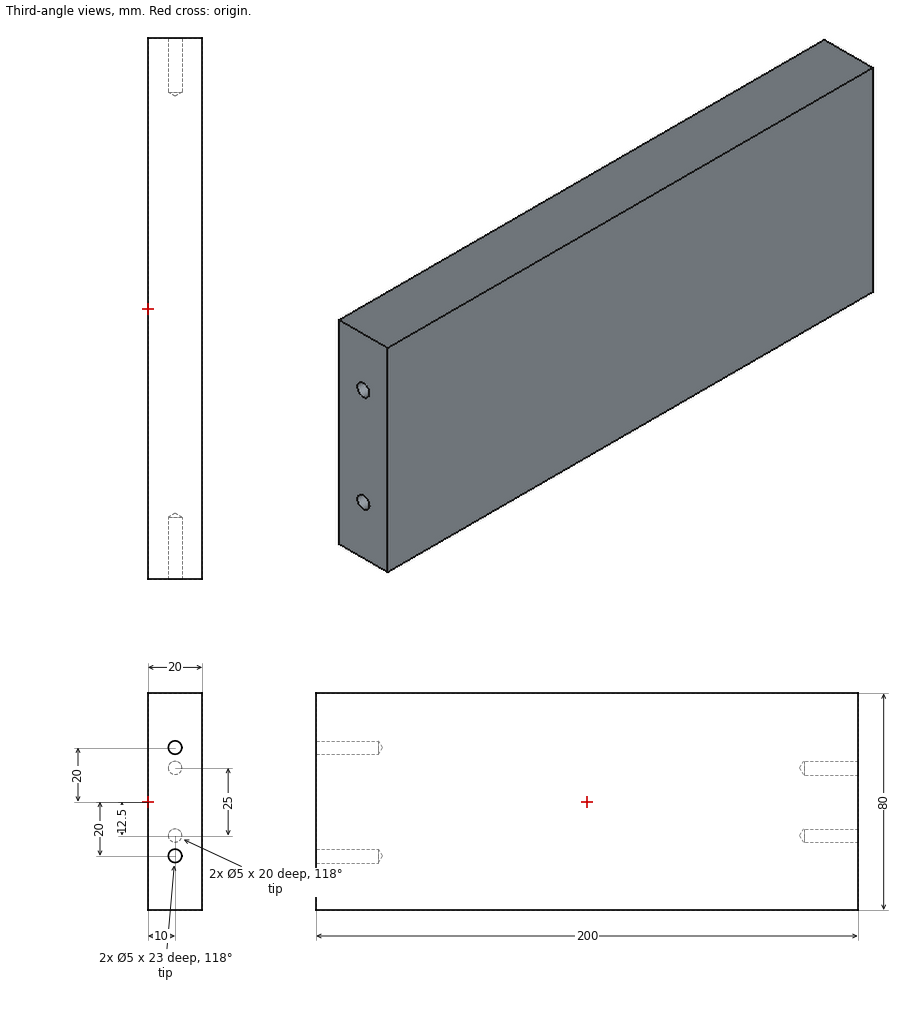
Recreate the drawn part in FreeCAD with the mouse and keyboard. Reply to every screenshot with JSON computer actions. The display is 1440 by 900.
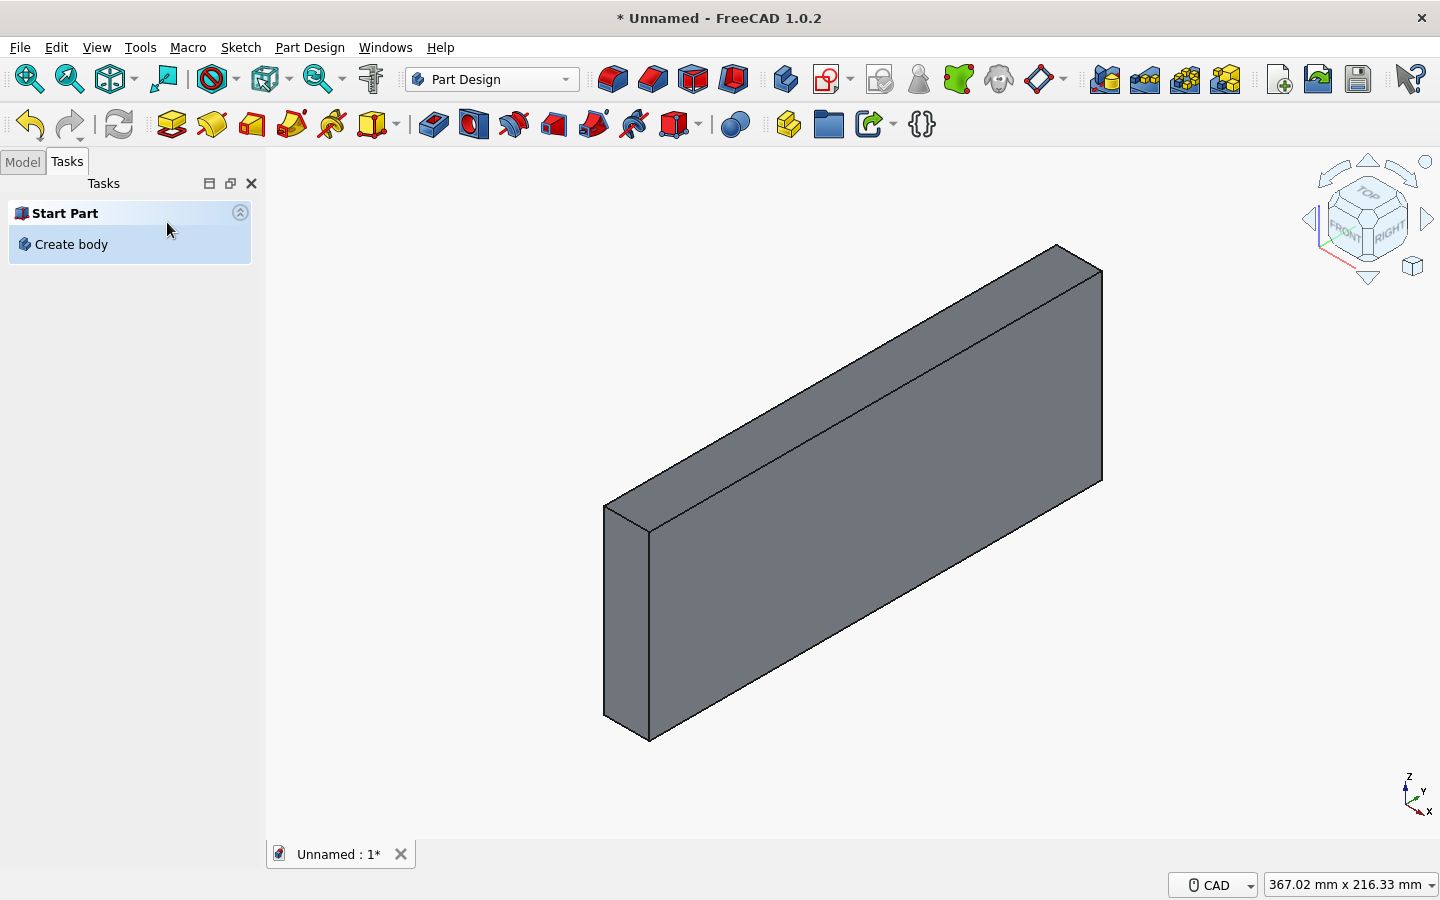
{"action": "left_click", "coordinate": [627, 652]}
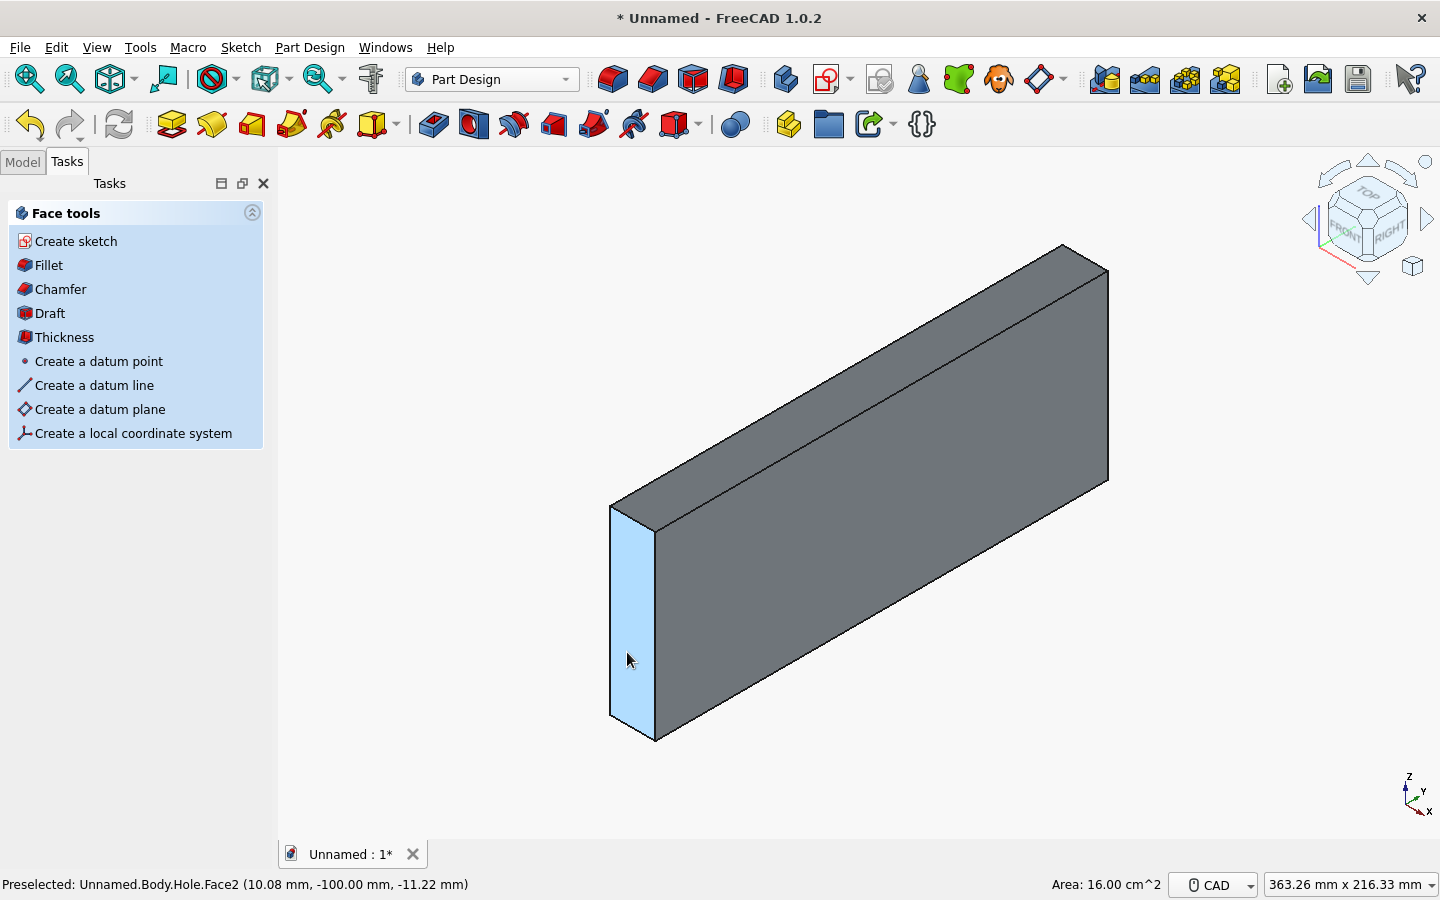
{"action": "left_click", "coordinate": [826, 80]}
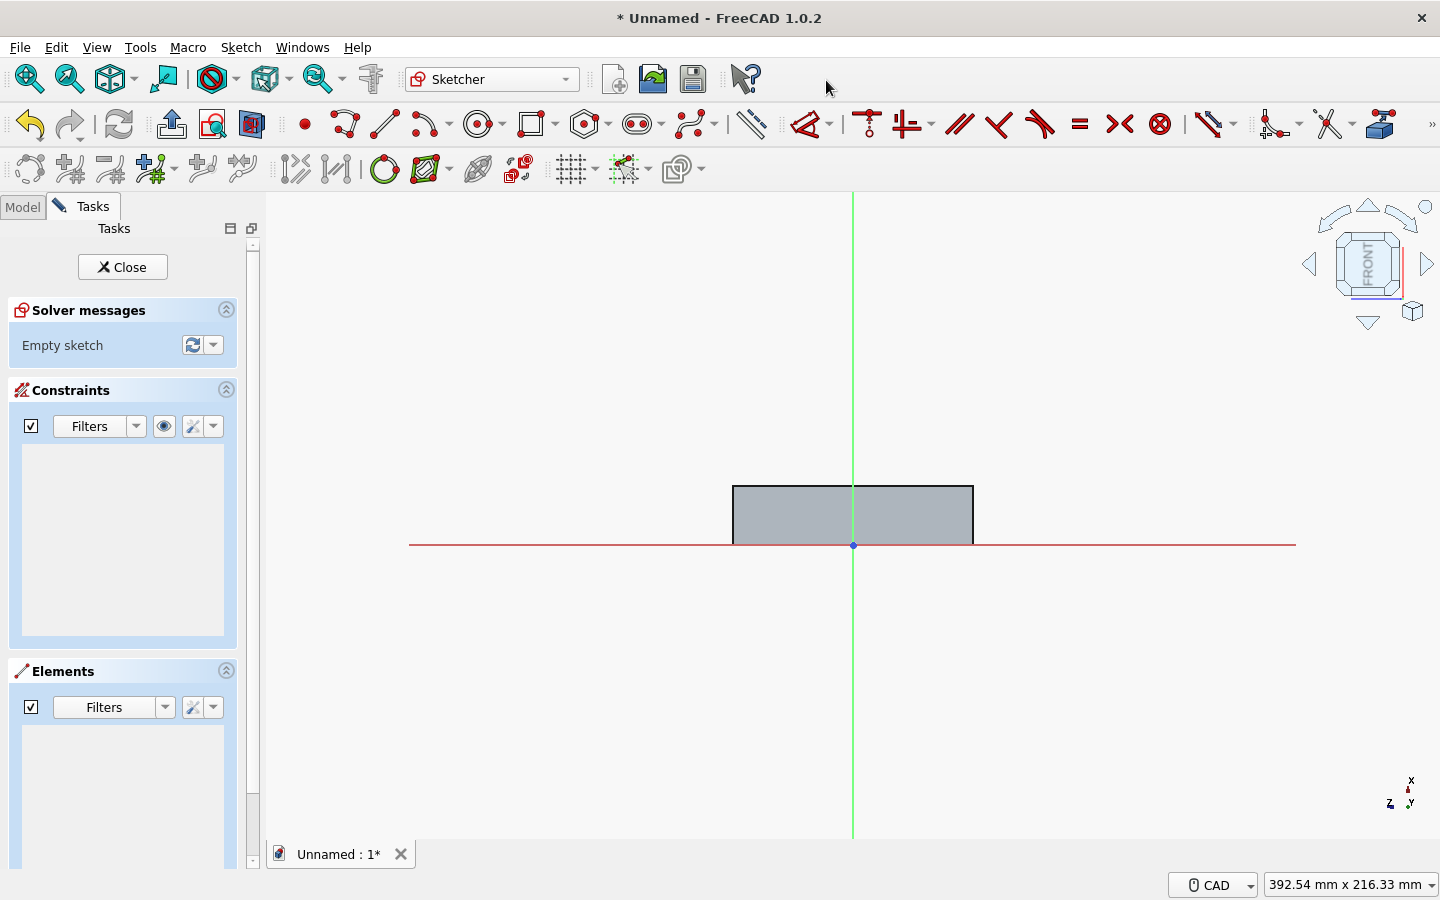
{"action": "scroll", "coordinate": [870, 530], "scroll_direction": "up", "scroll_amount": 8}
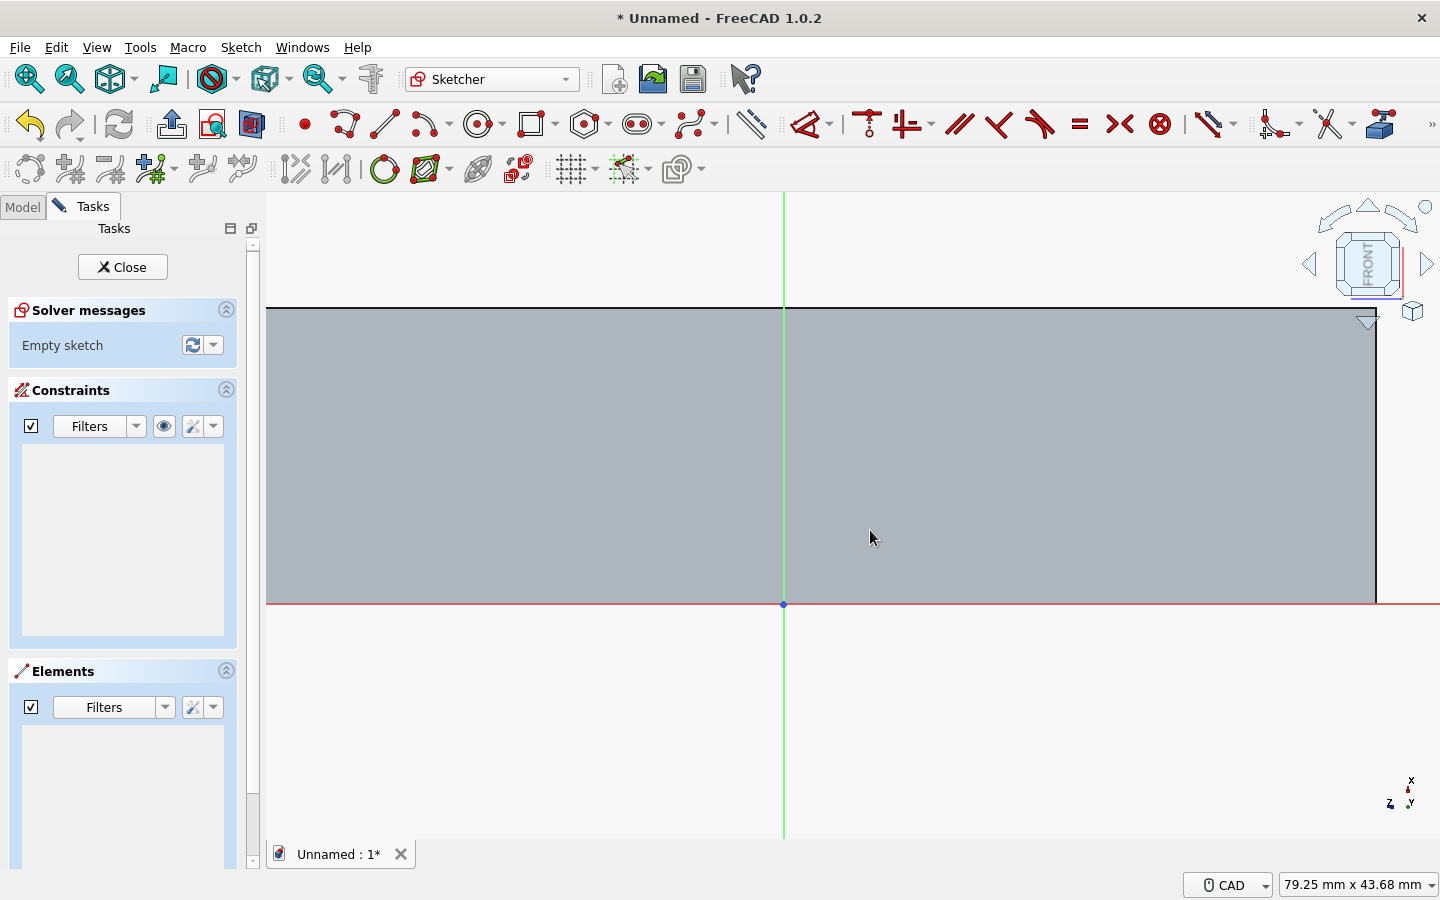
{"action": "key", "text": "g c"}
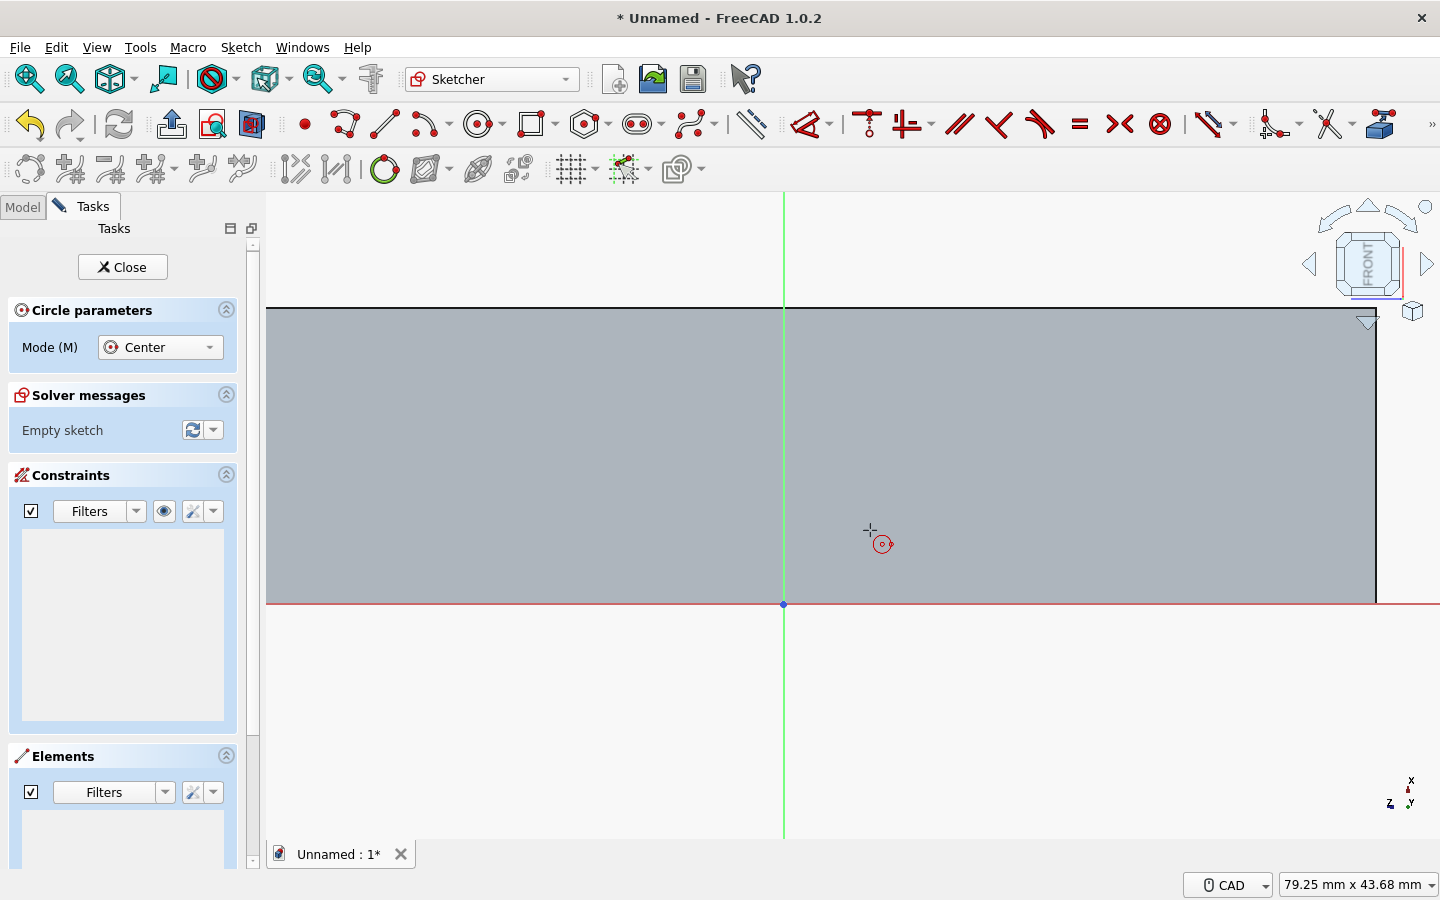
{"action": "left_click", "coordinate": [1080, 456]}
{"action": "mouse_move", "coordinate": [1106, 430]}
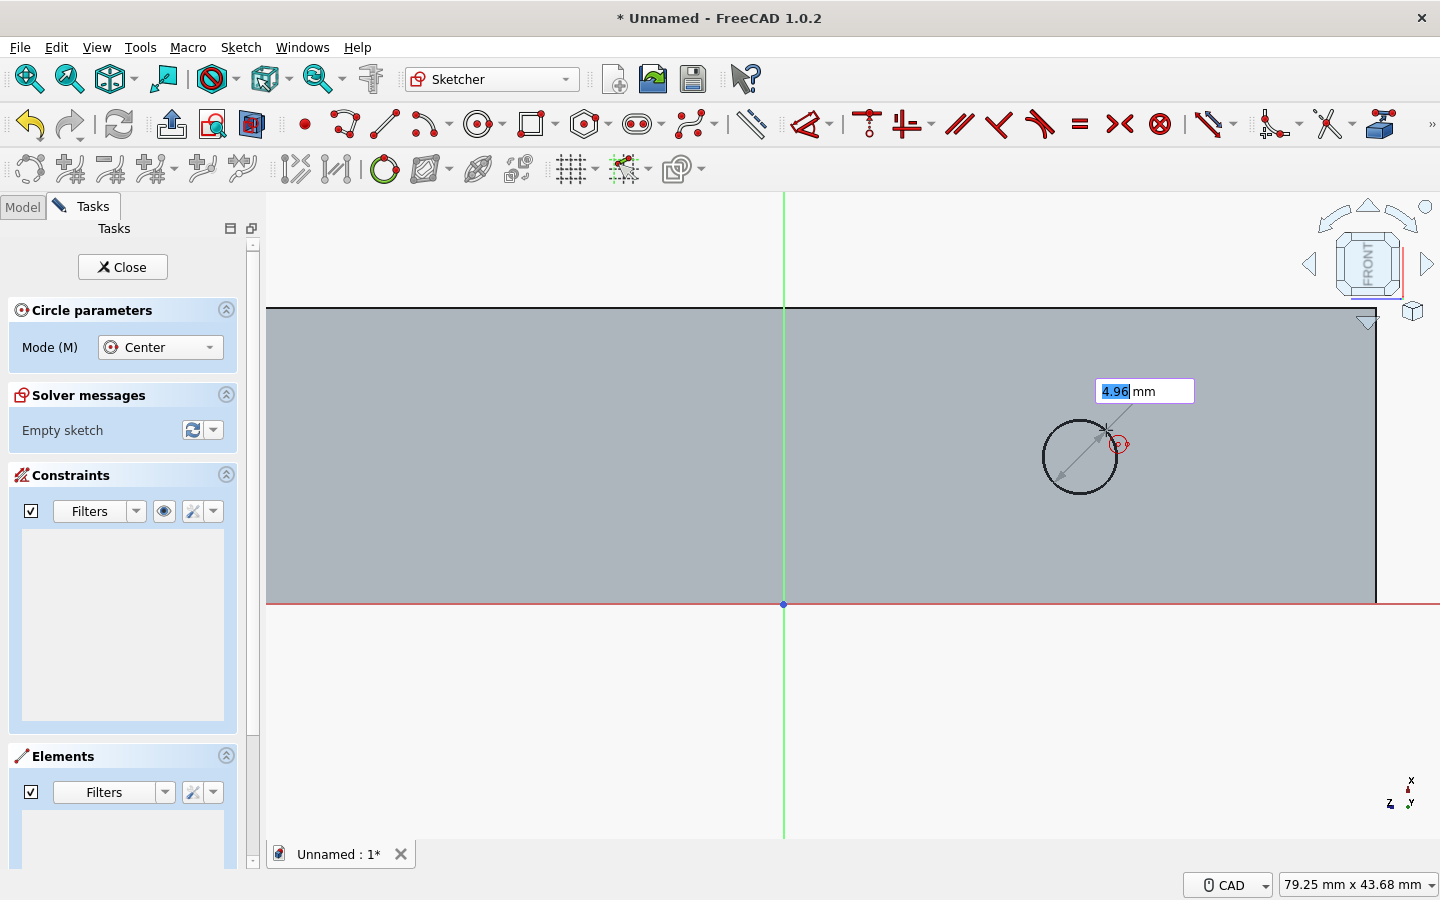
{"action": "type", "text": "5"}
{"action": "key", "text": "Return"}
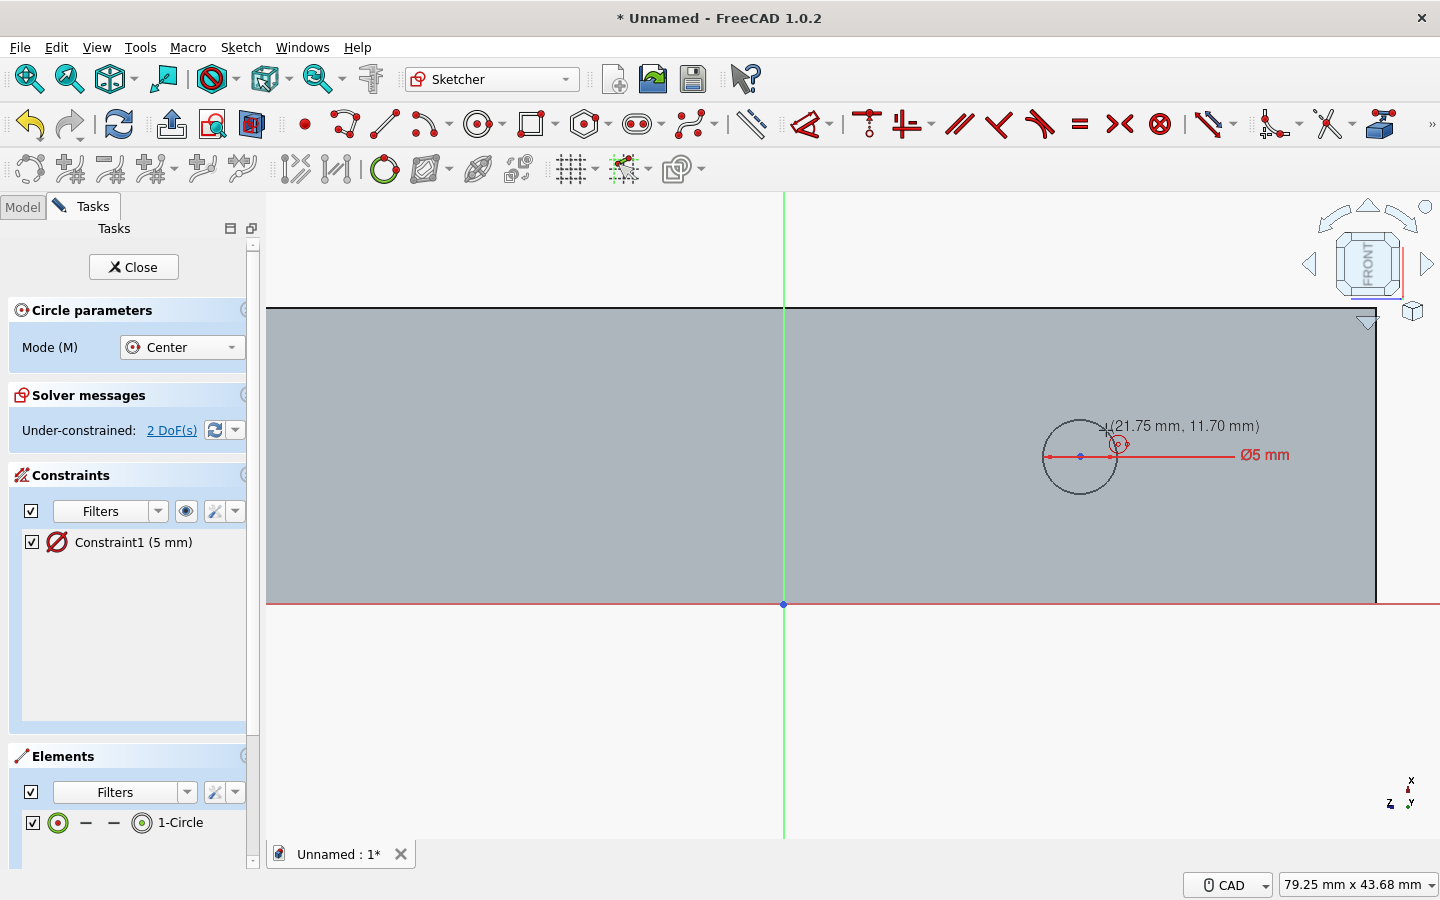
{"action": "left_click", "coordinate": [487, 456]}
{"action": "mouse_move", "coordinate": [514, 430]}